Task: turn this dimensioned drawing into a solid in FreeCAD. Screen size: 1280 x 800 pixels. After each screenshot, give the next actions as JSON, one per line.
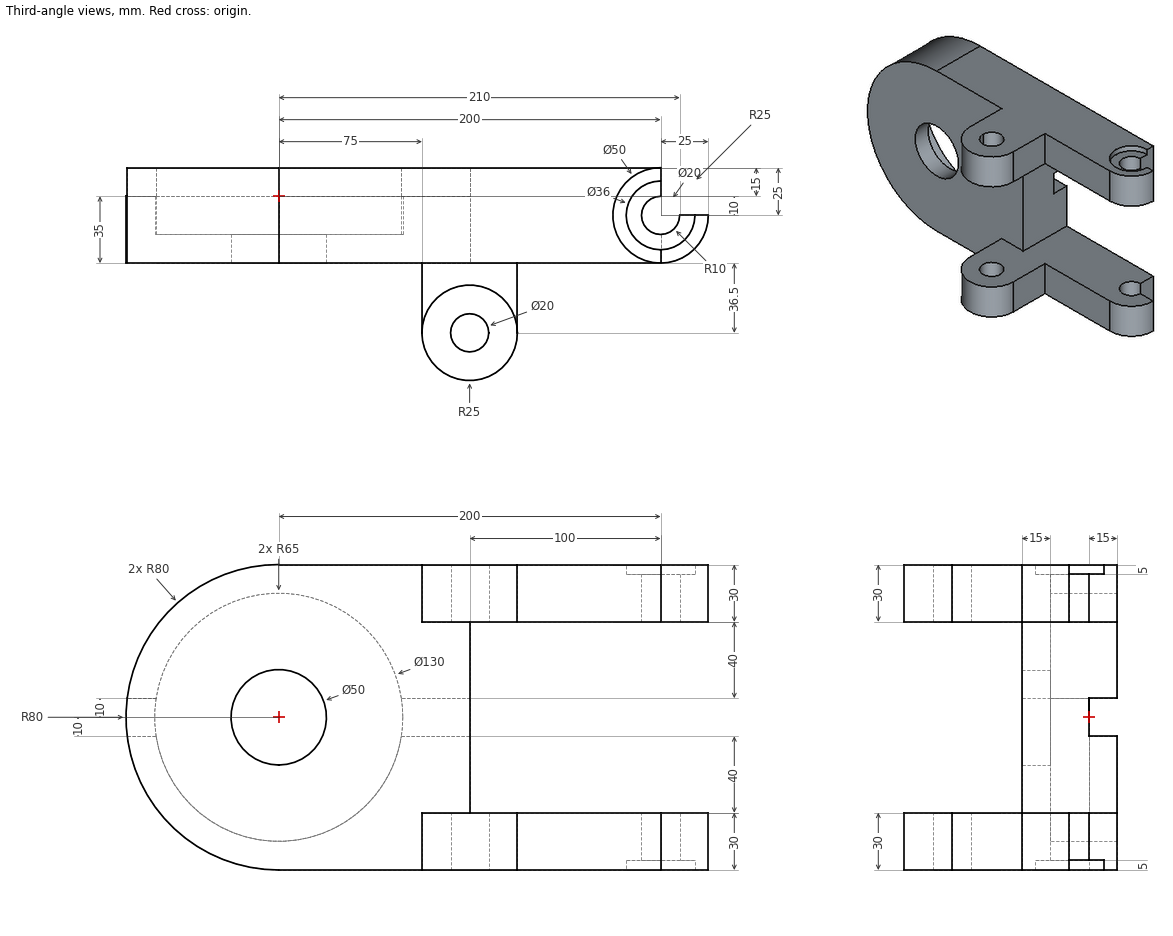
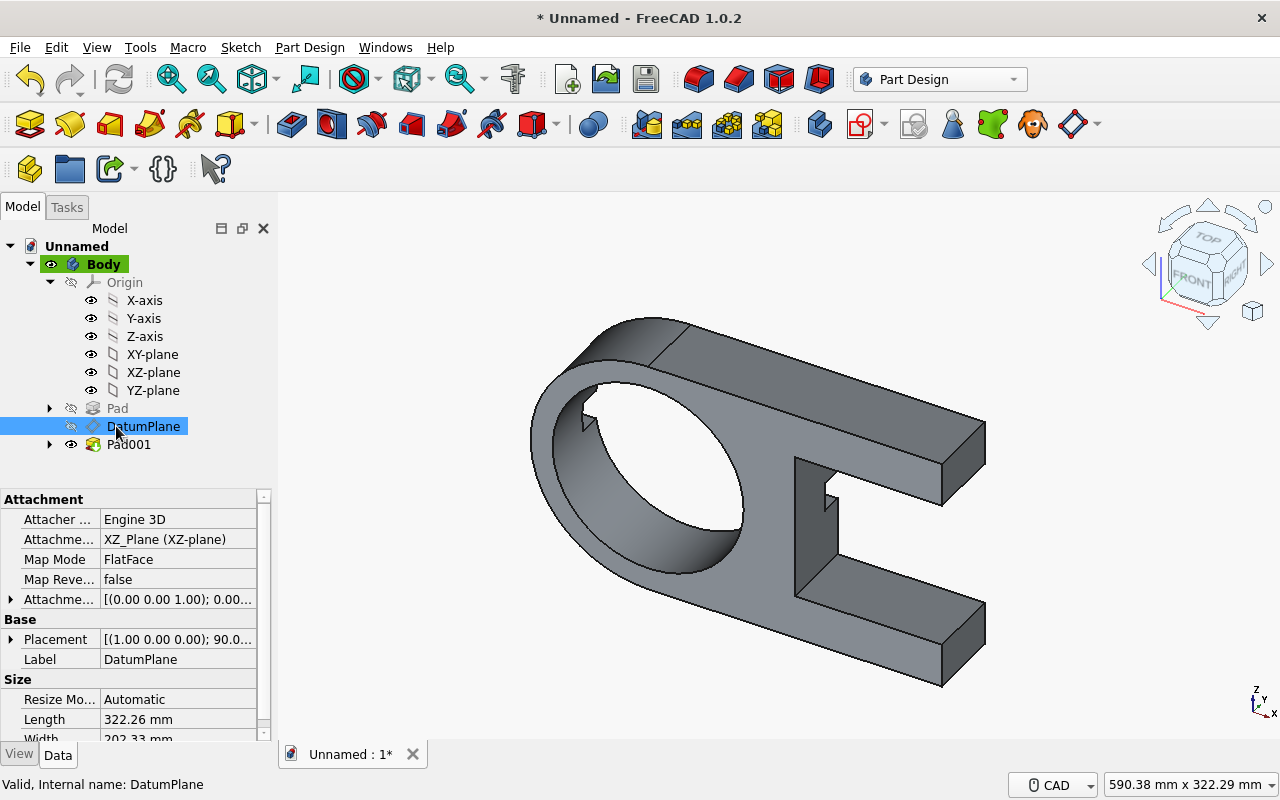
{"action": "left_click", "coordinate": [913, 660]}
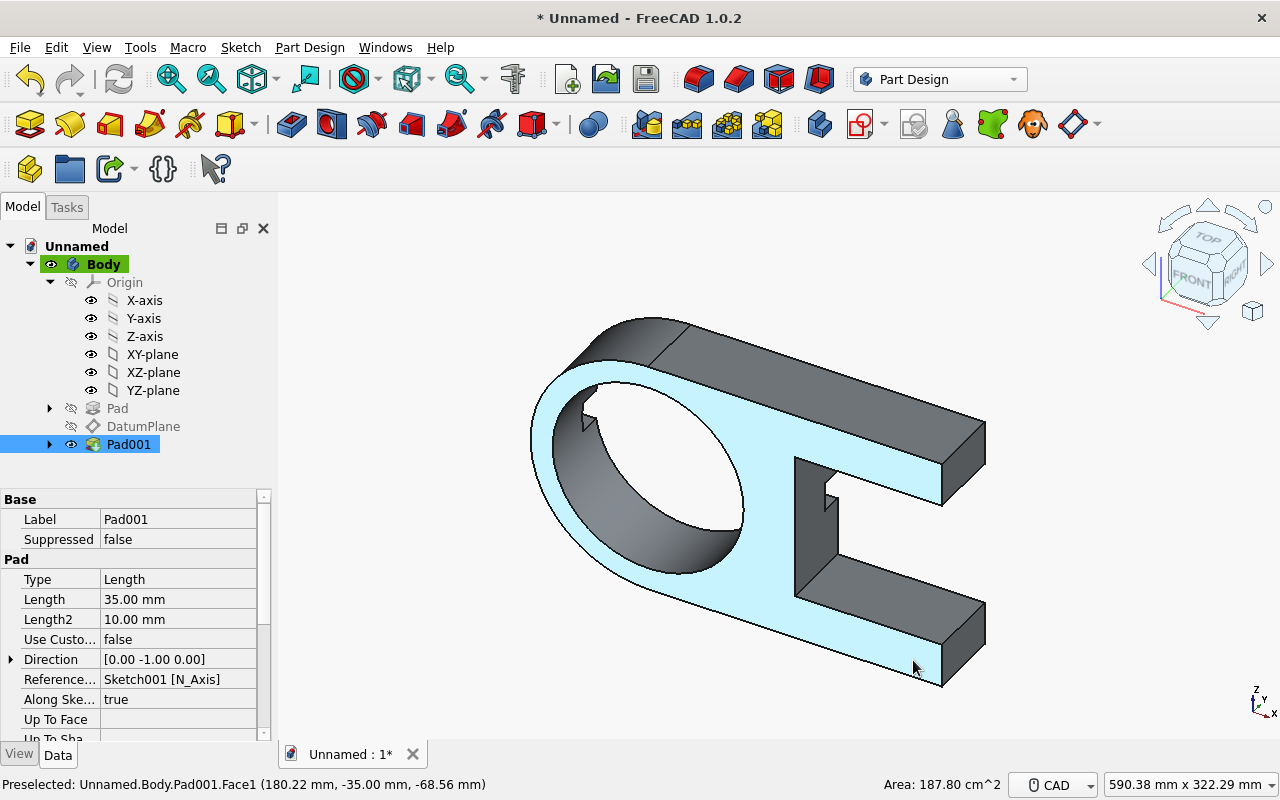
{"action": "left_click", "coordinate": [860, 124]}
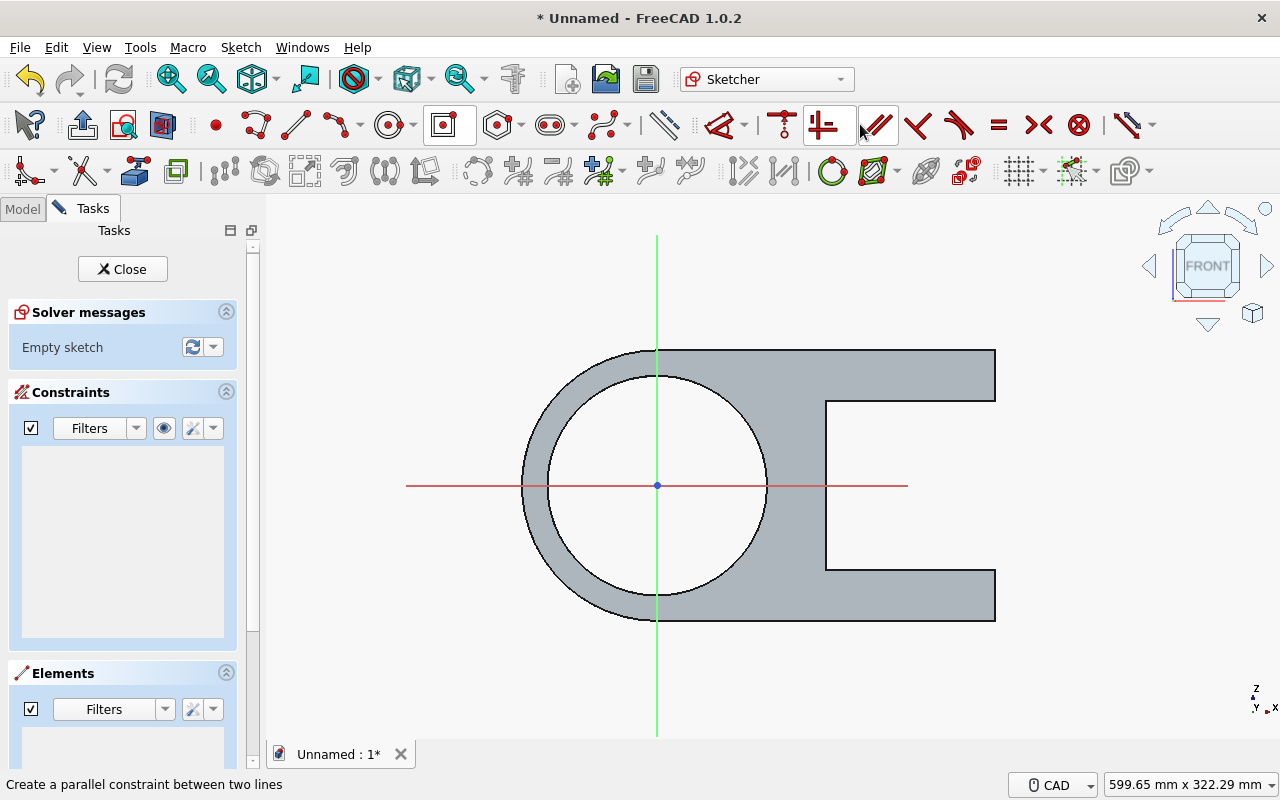
{"action": "scroll", "coordinate": [561, 525], "scroll_direction": "up", "scroll_amount": 2}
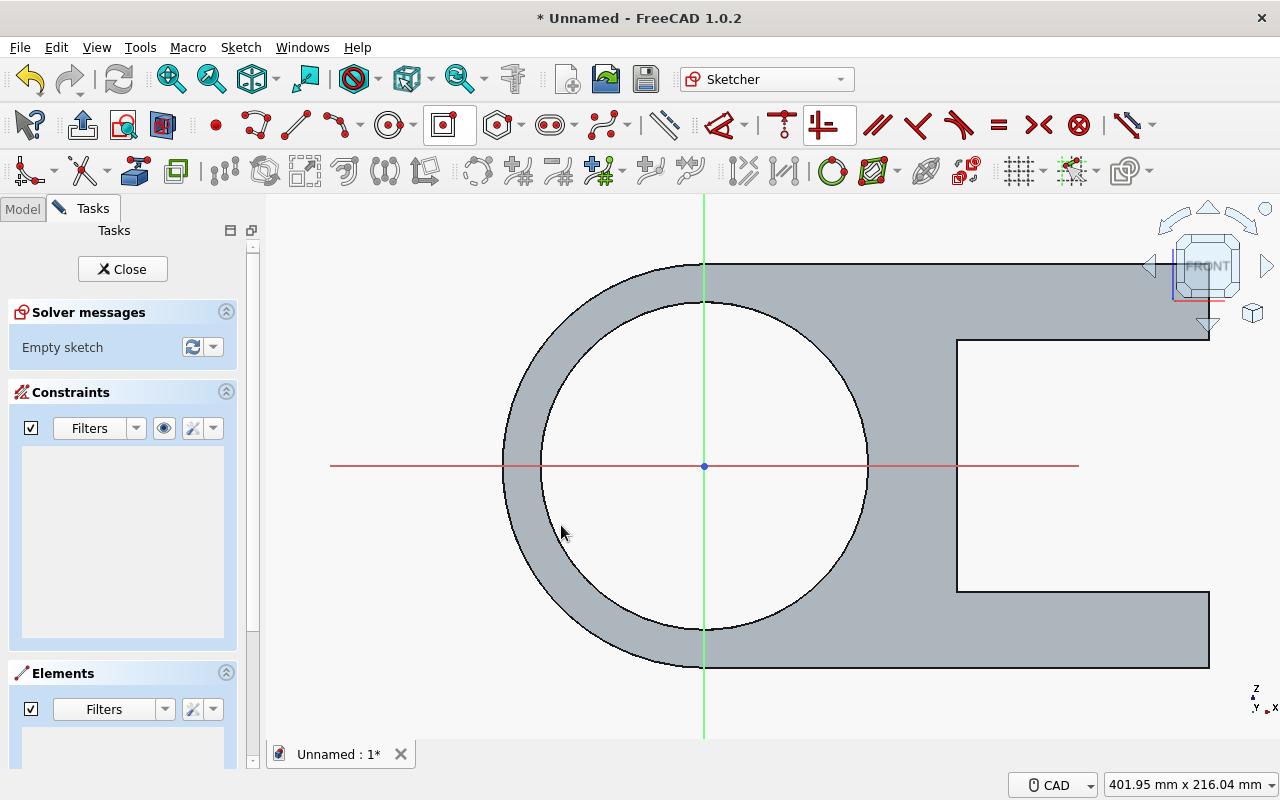
{"action": "left_click", "coordinate": [390, 126]}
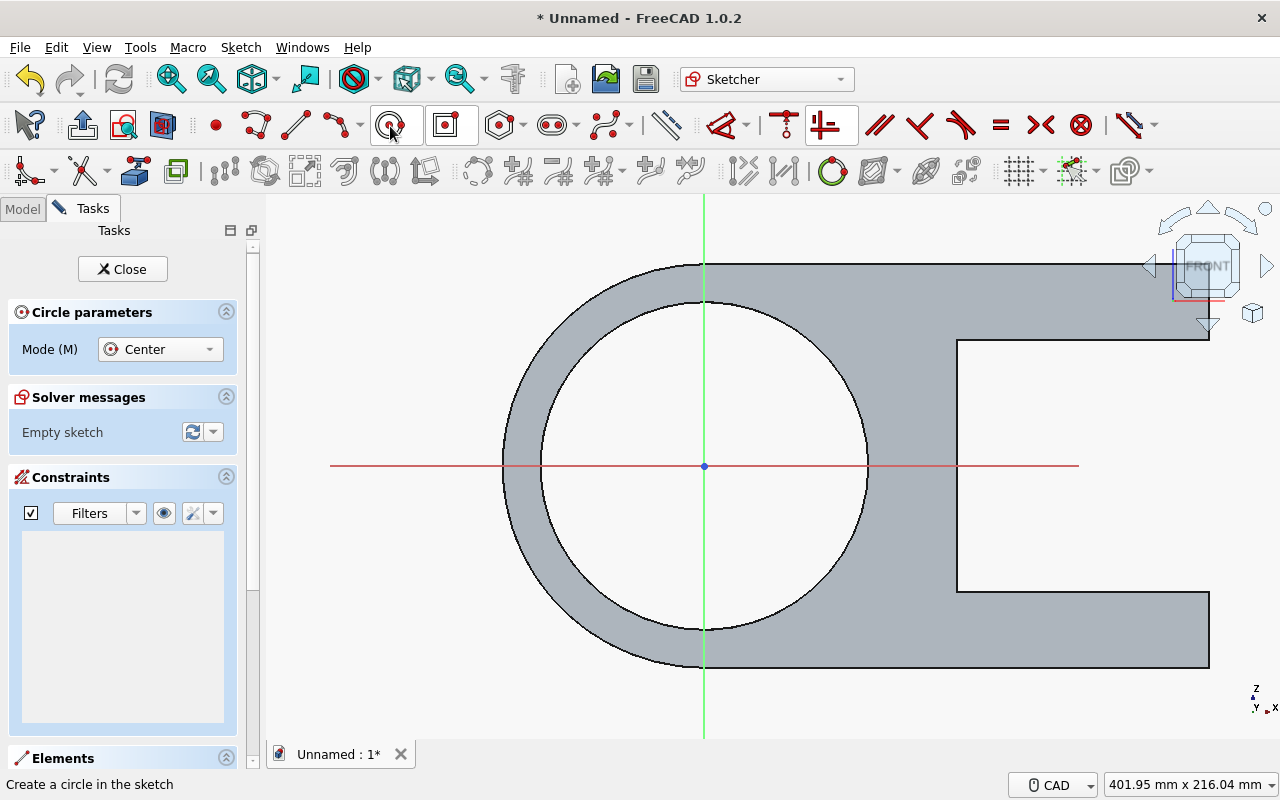
{"action": "left_click", "coordinate": [704, 466]}
{"action": "left_click", "coordinate": [820, 350]}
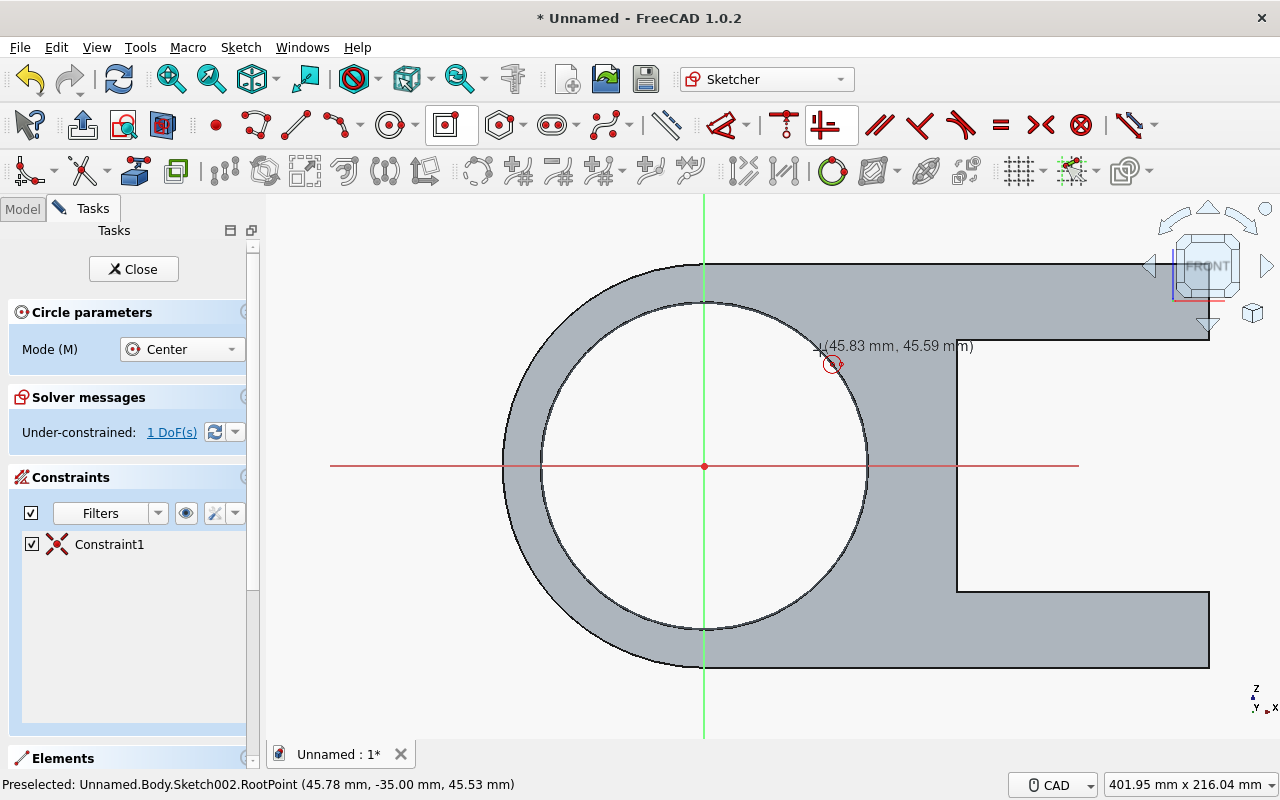
{"action": "left_click", "coordinate": [704, 466]}
{"action": "left_click", "coordinate": [749, 421]}
{"action": "key", "text": "Escape"}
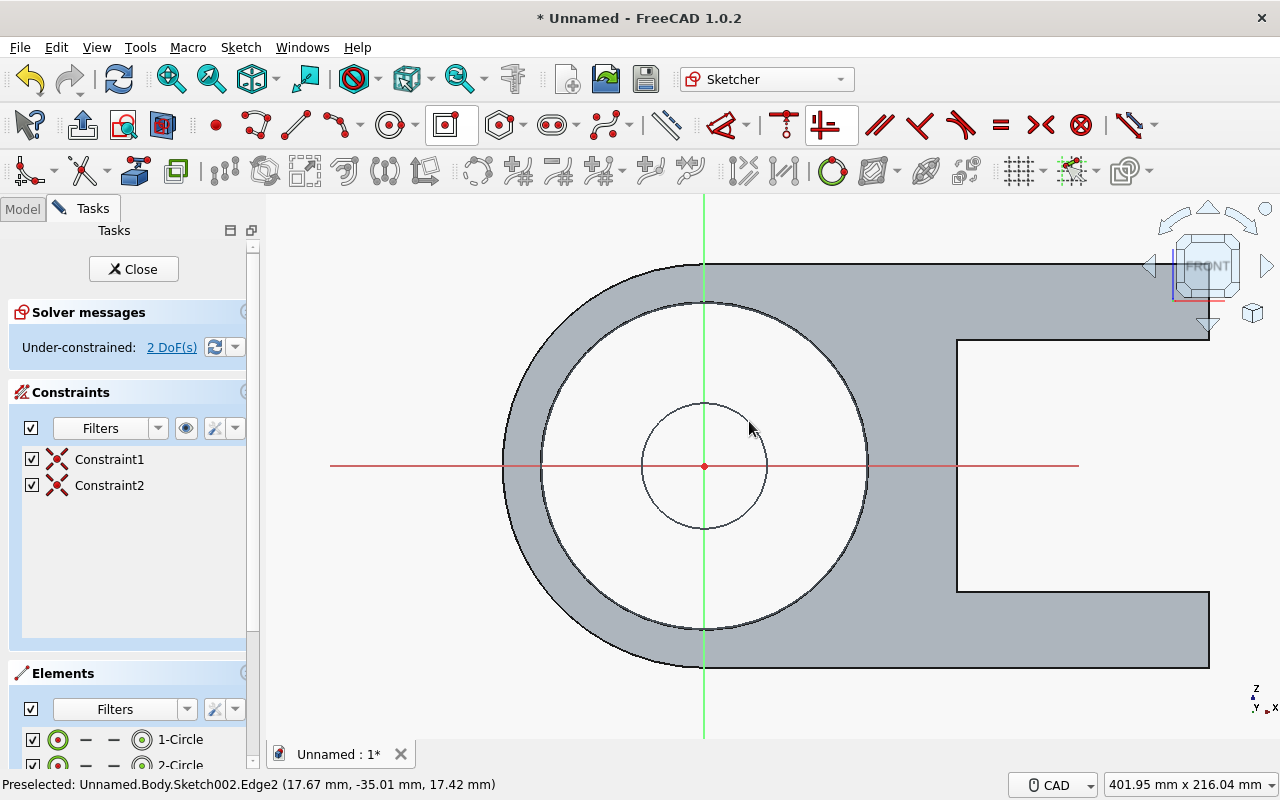
{"action": "left_click", "coordinate": [722, 126]}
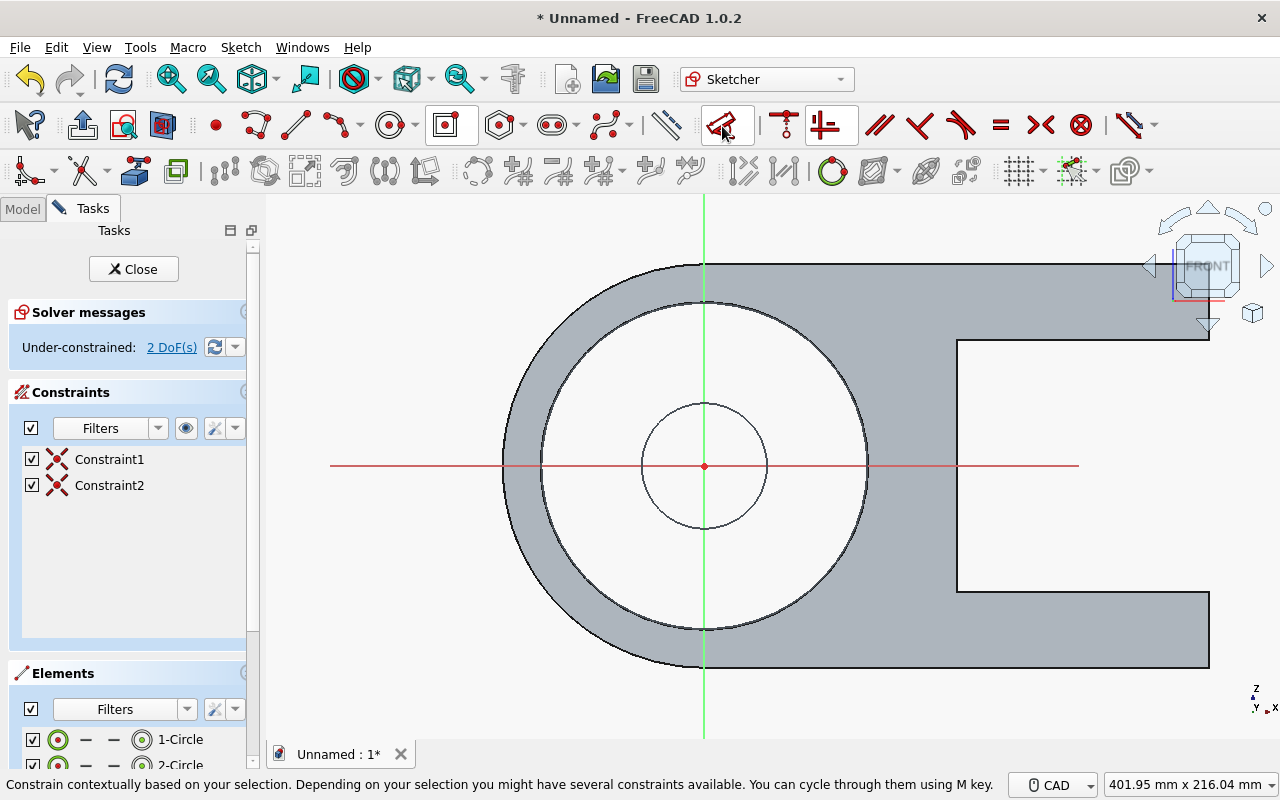
{"action": "left_click", "coordinate": [819, 350]}
{"action": "left_click", "coordinate": [841, 327]}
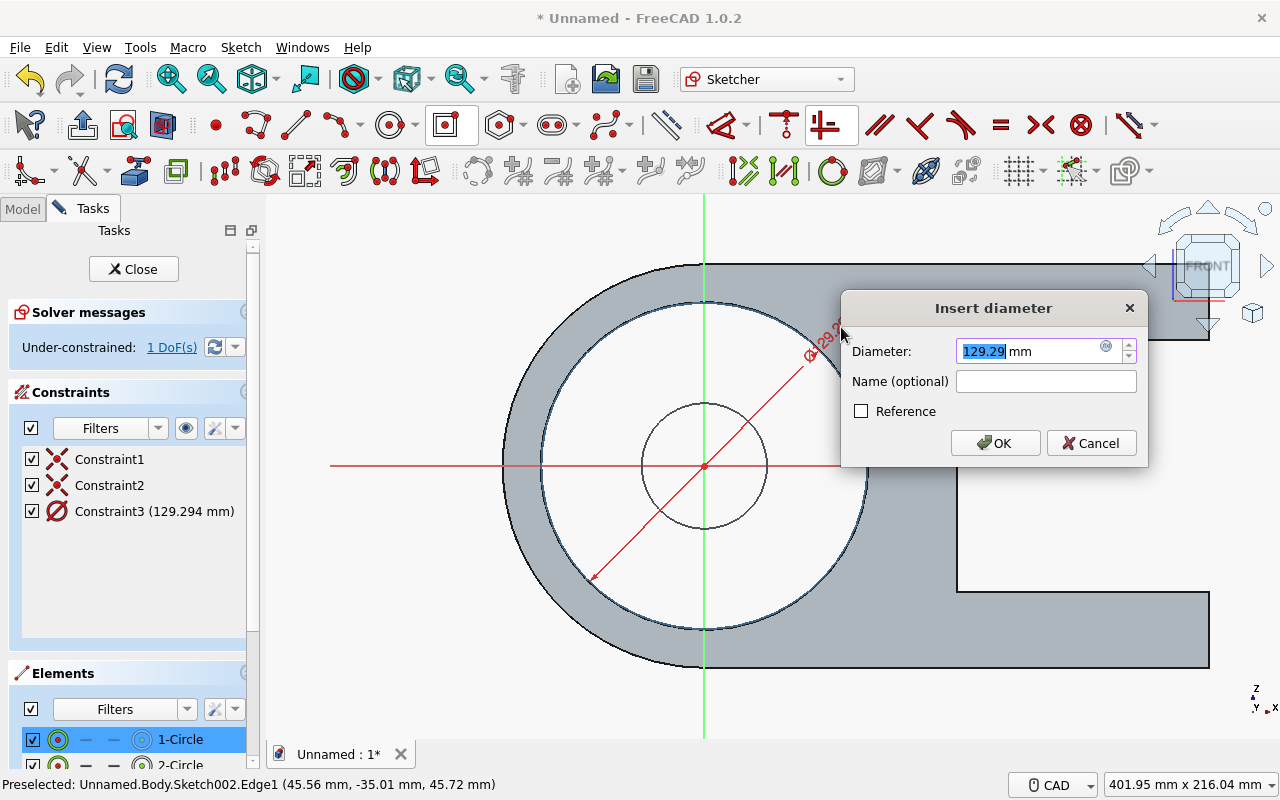
{"action": "type", "text": "130"}
{"action": "key", "text": "Return"}